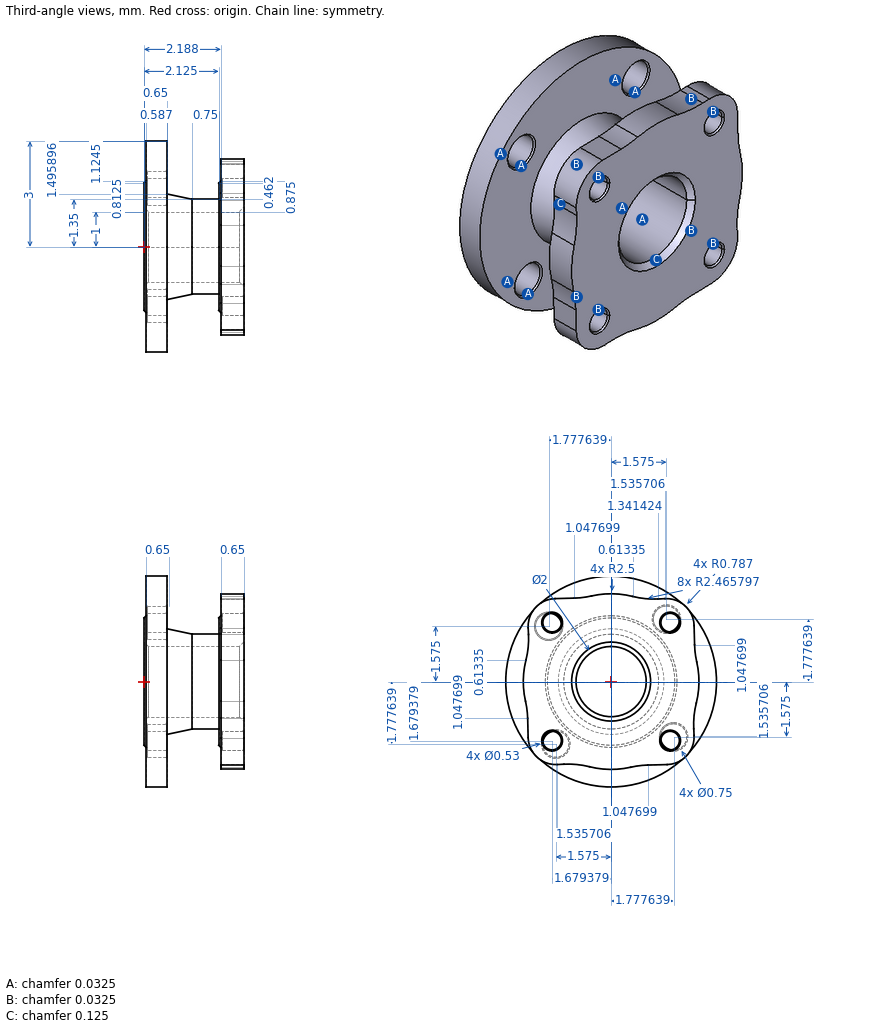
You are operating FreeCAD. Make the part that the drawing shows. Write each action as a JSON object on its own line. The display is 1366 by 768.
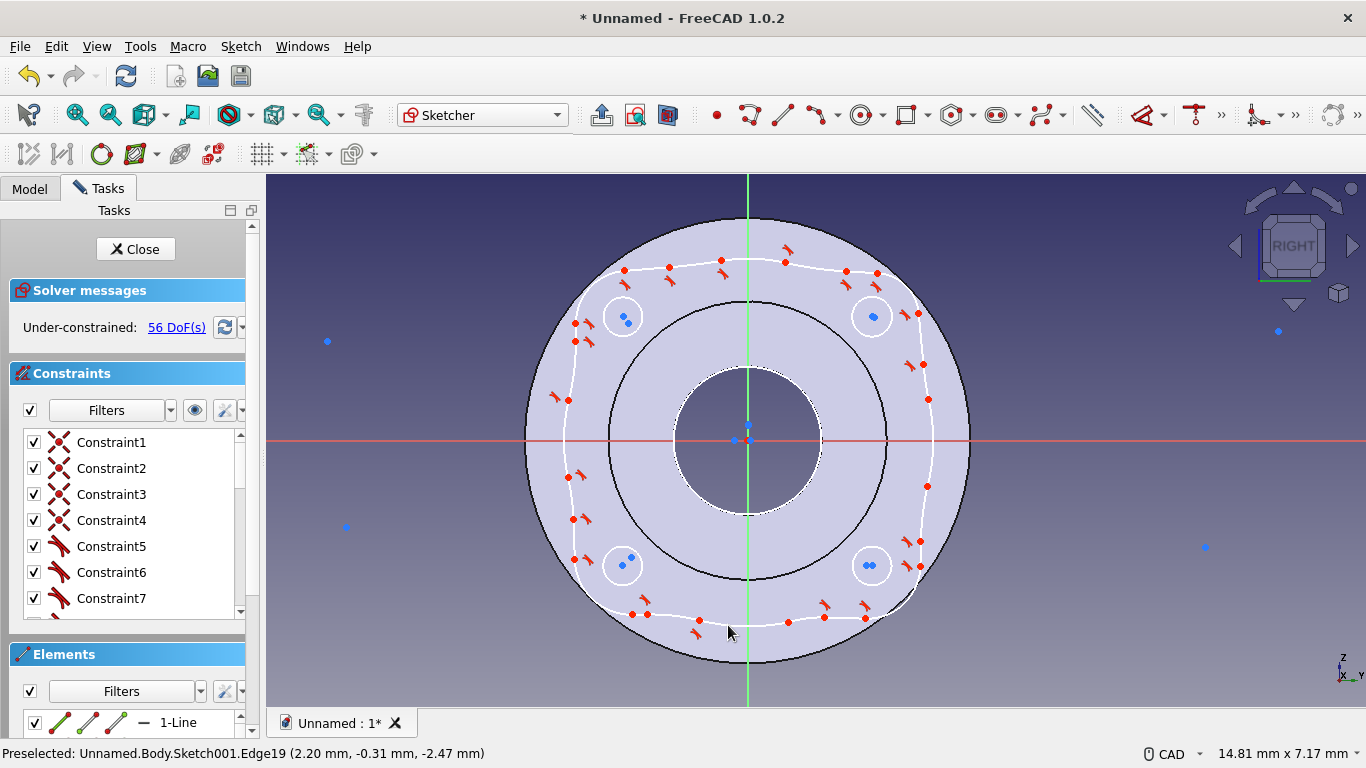
{"action": "left_click", "coordinate": [726, 625]}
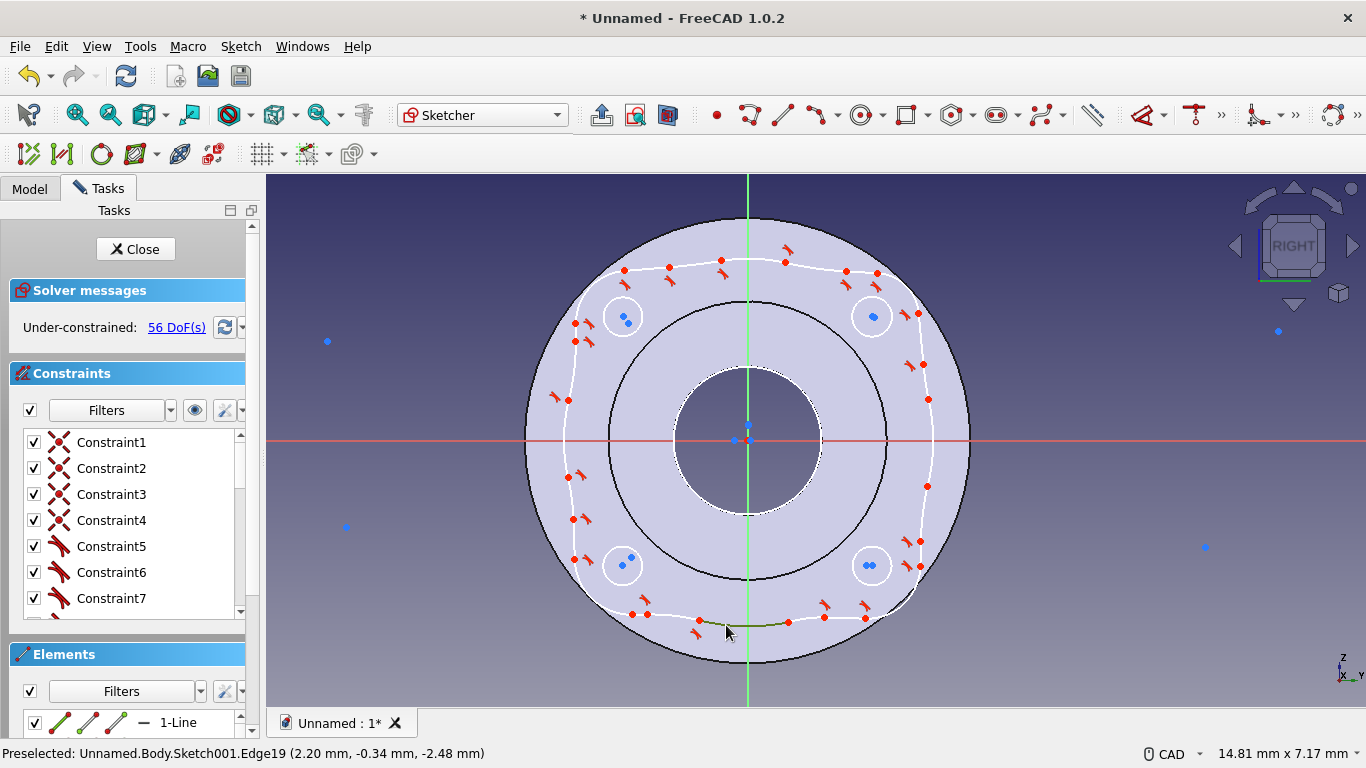
{"action": "scroll", "coordinate": [814, 618], "scroll_direction": "up", "scroll_amount": 2}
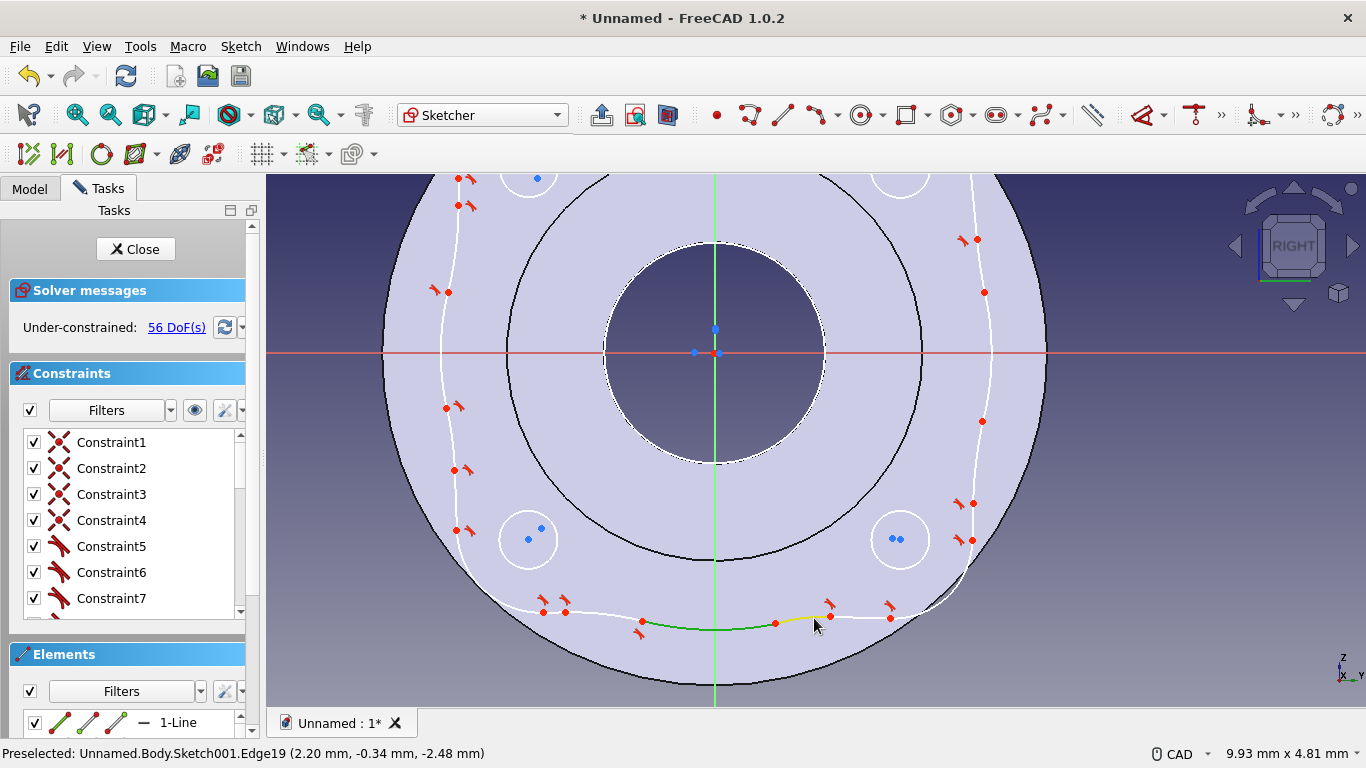
{"action": "left_click", "coordinate": [814, 617]}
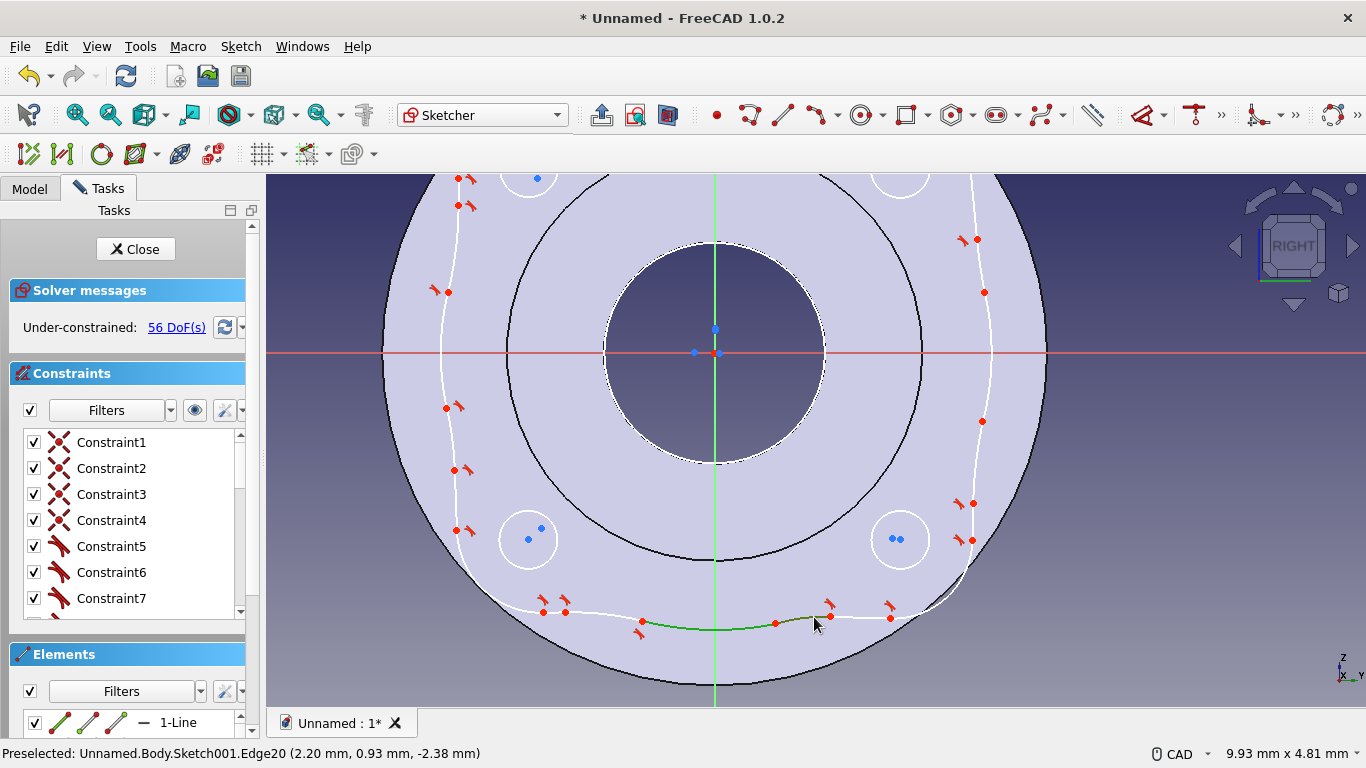
{"action": "key", "text": "t"}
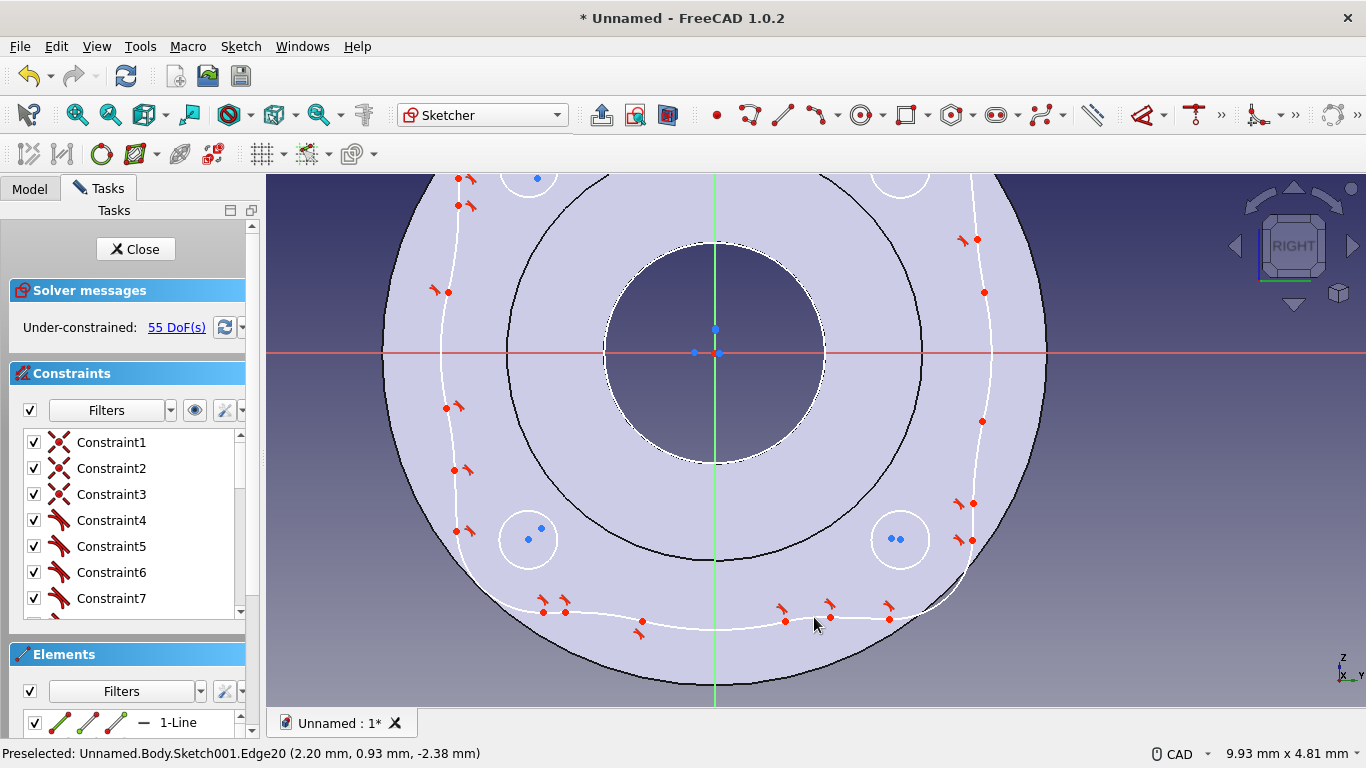
{"action": "left_click", "coordinate": [978, 446]}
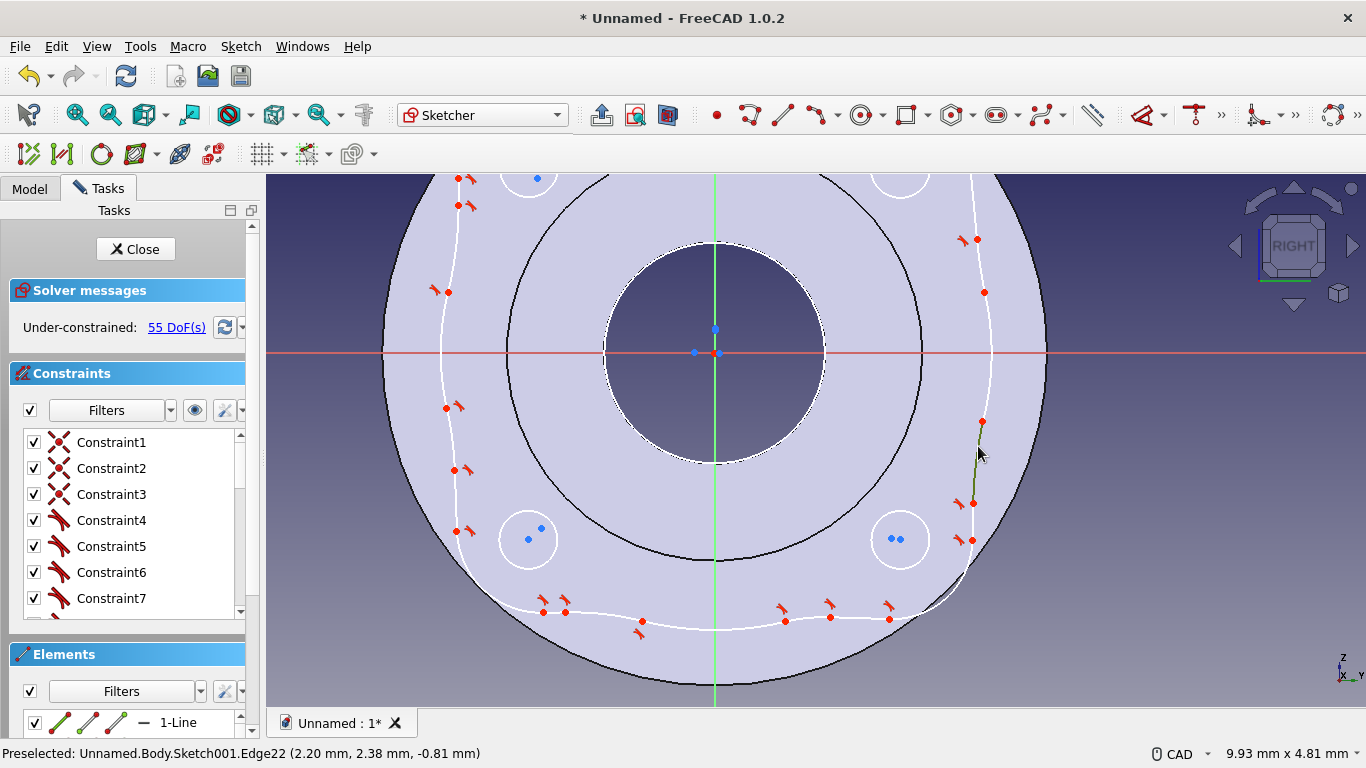
{"action": "left_click", "coordinate": [990, 383]}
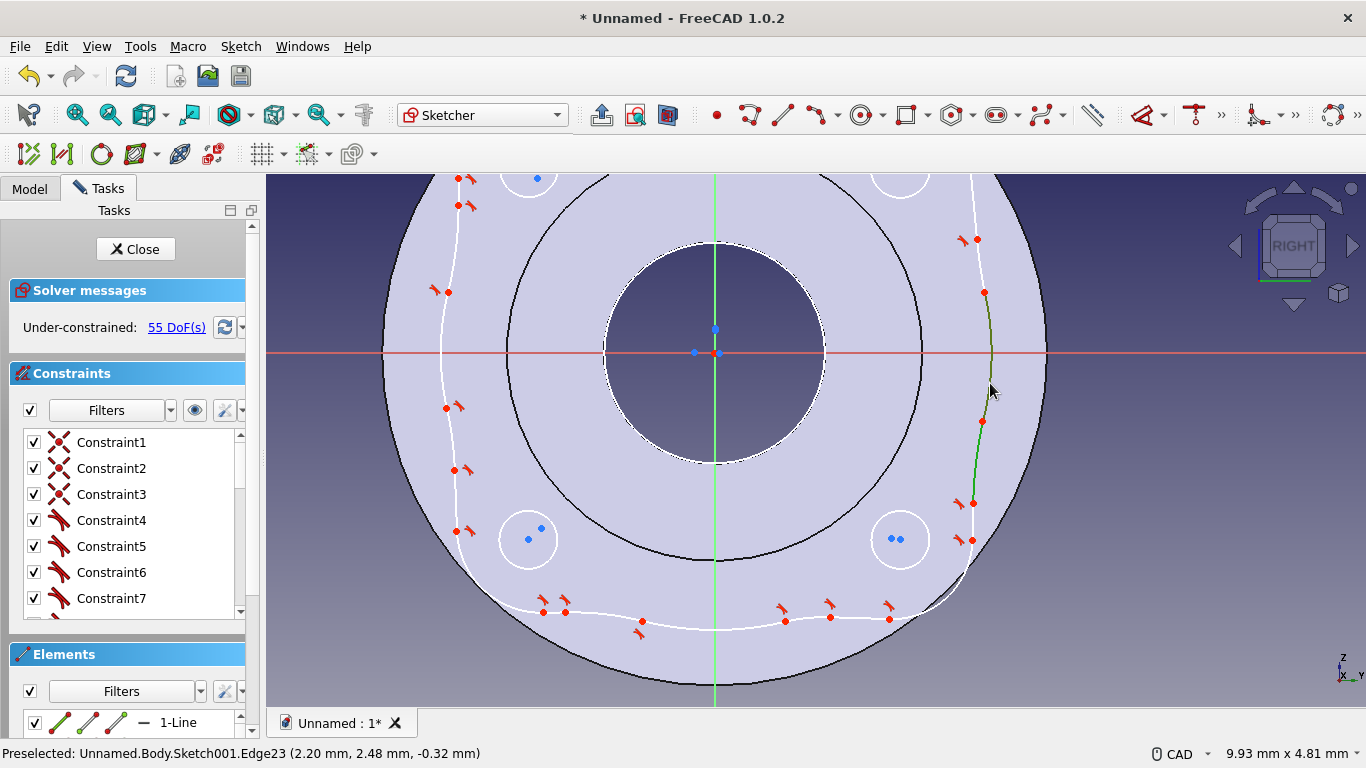
{"action": "key", "text": "t"}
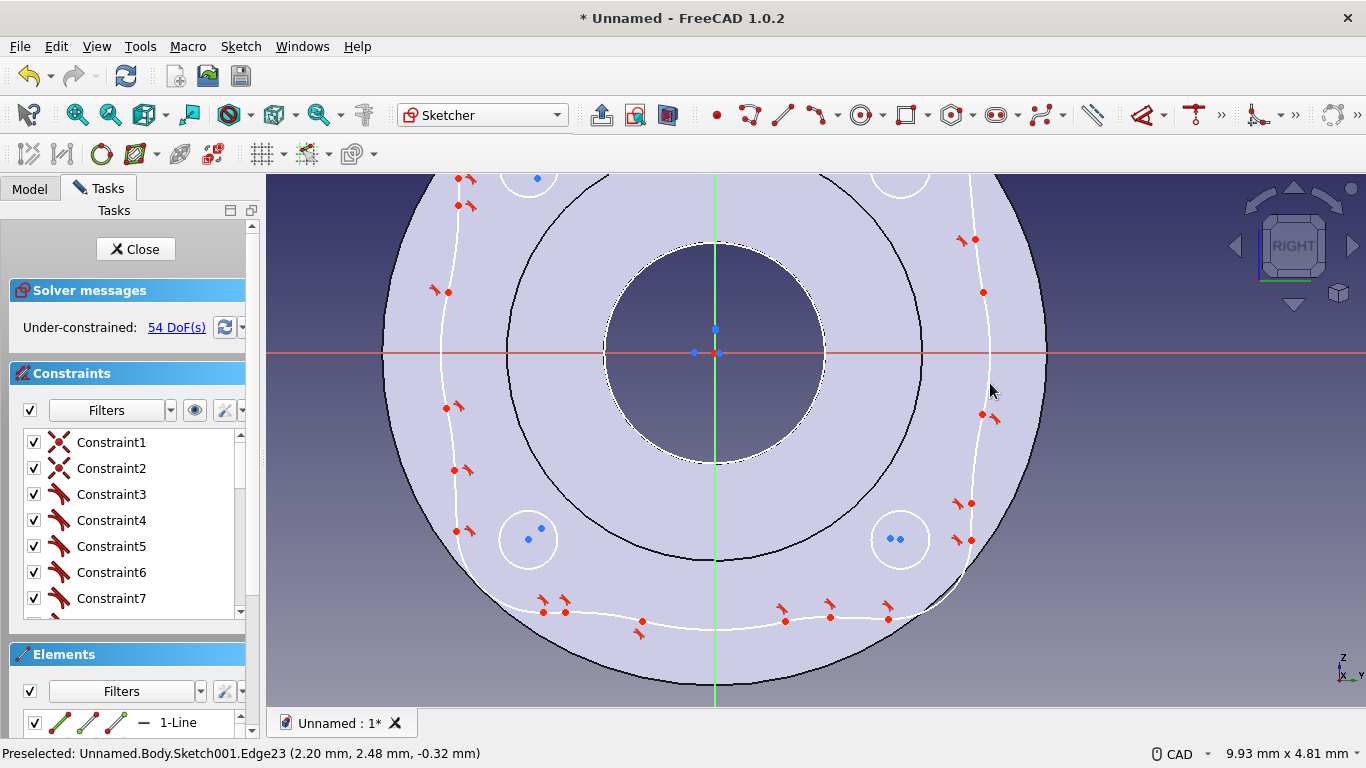
{"action": "left_click", "coordinate": [989, 378]}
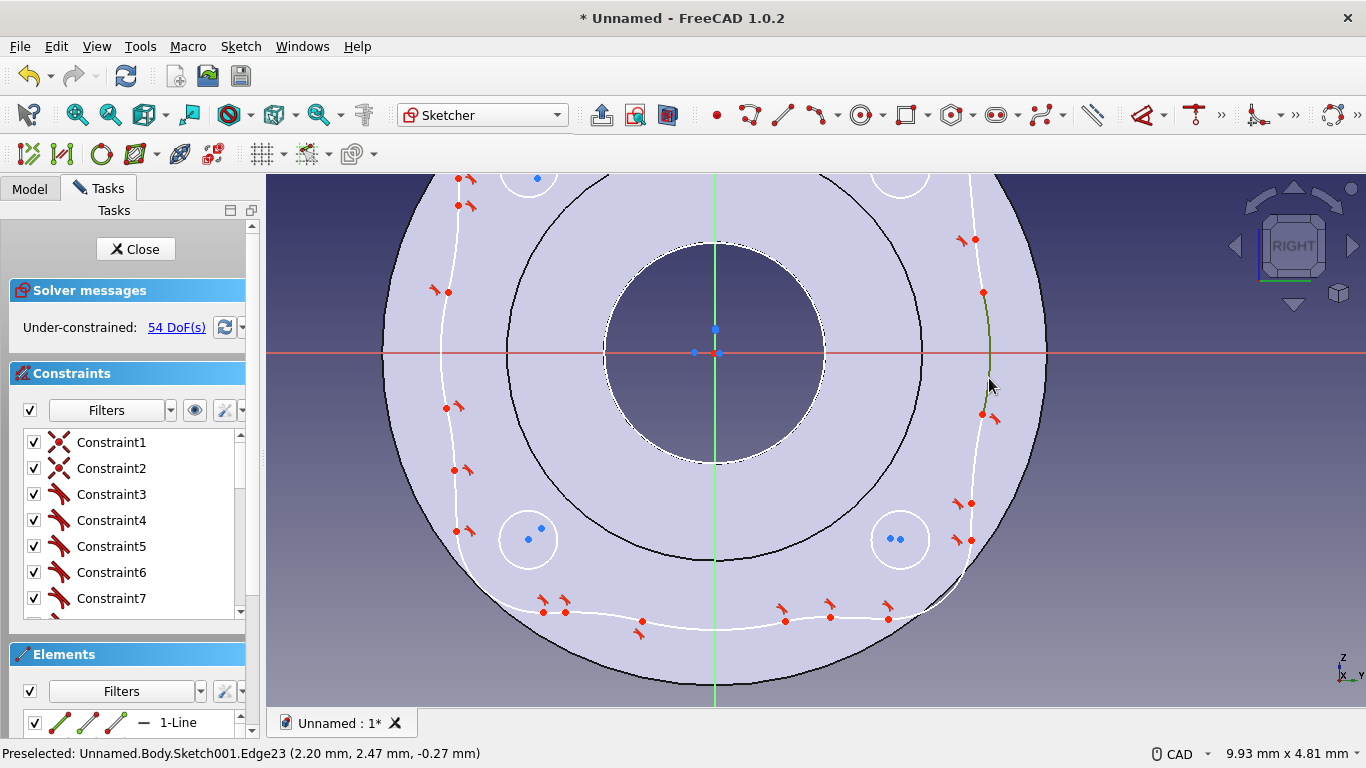
{"action": "left_click", "coordinate": [977, 255]}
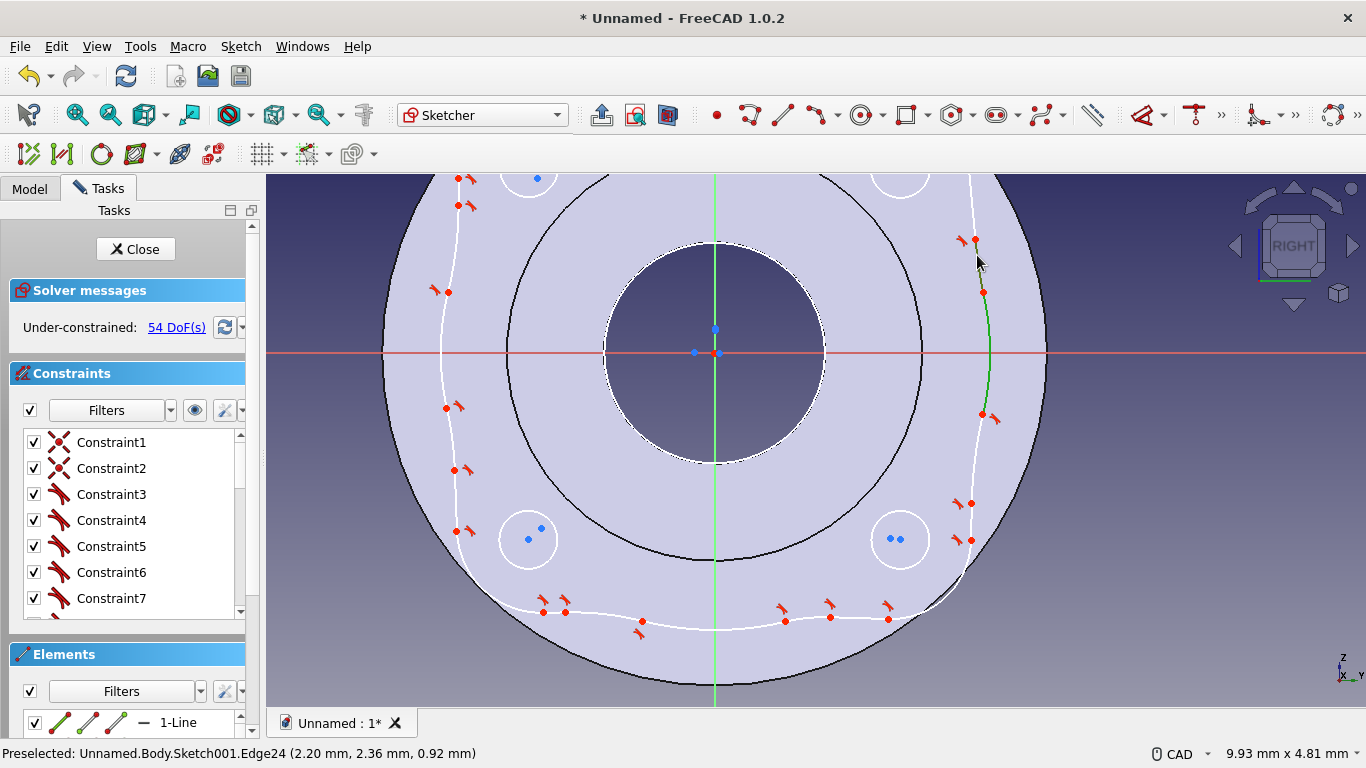
{"action": "key", "text": "t"}